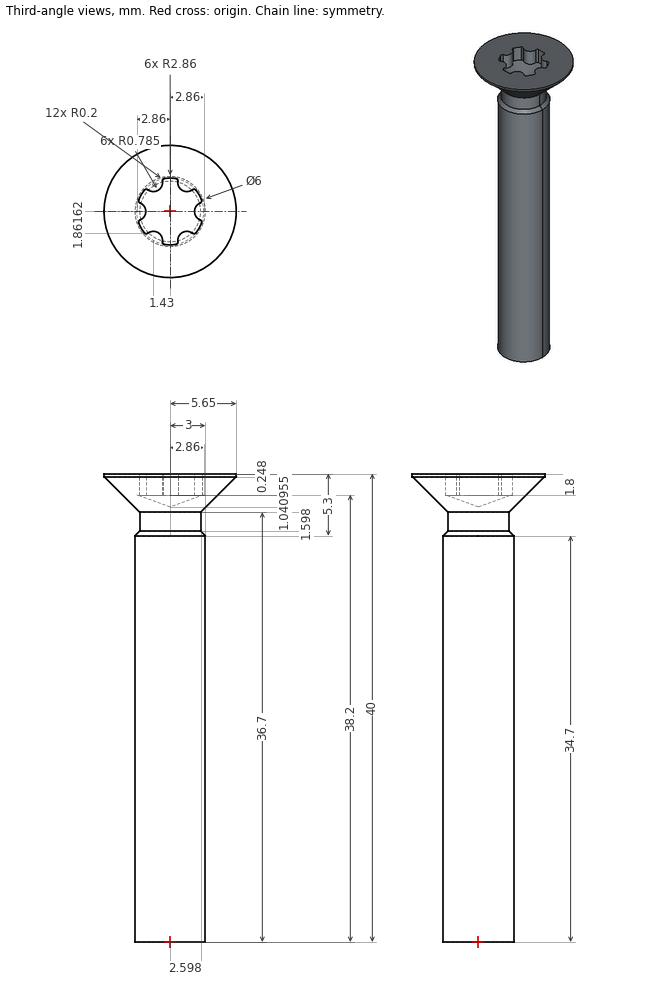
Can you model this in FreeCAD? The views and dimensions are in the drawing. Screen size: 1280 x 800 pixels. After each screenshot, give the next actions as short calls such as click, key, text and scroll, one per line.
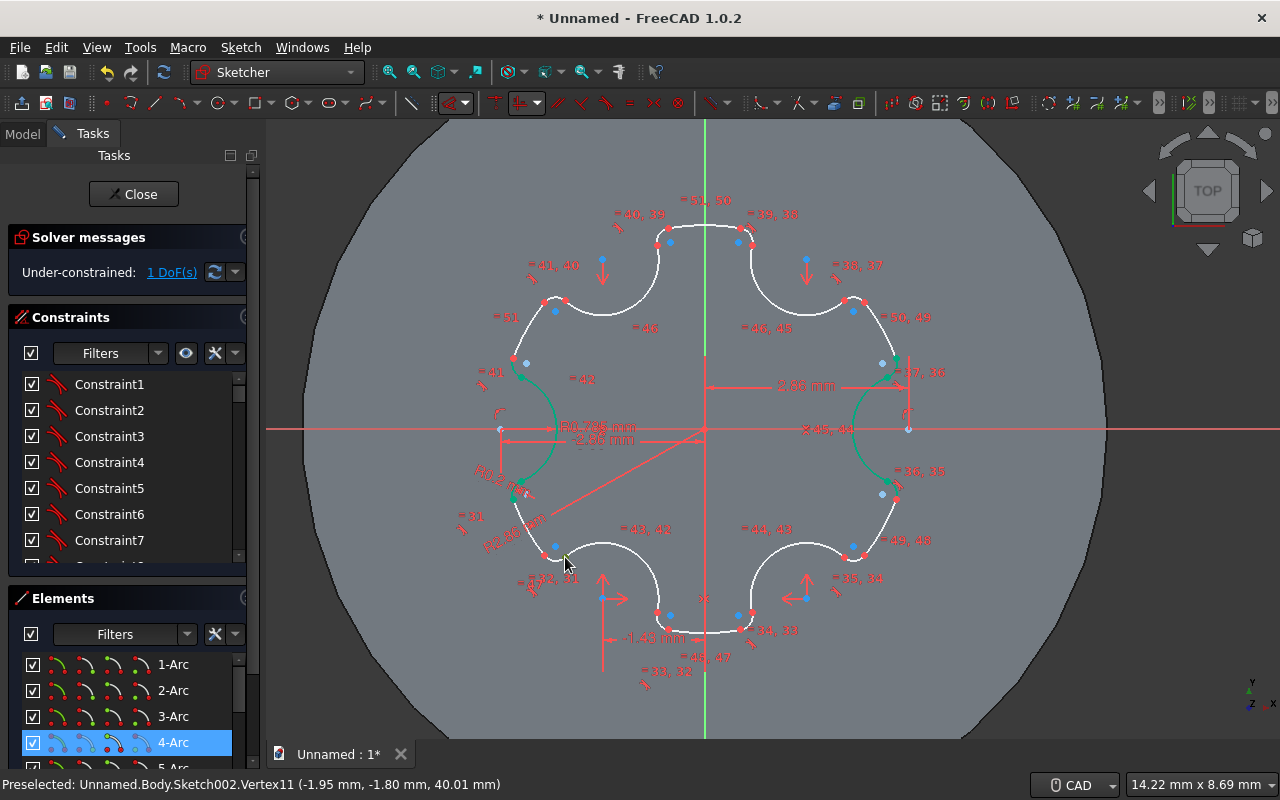
click(468, 104)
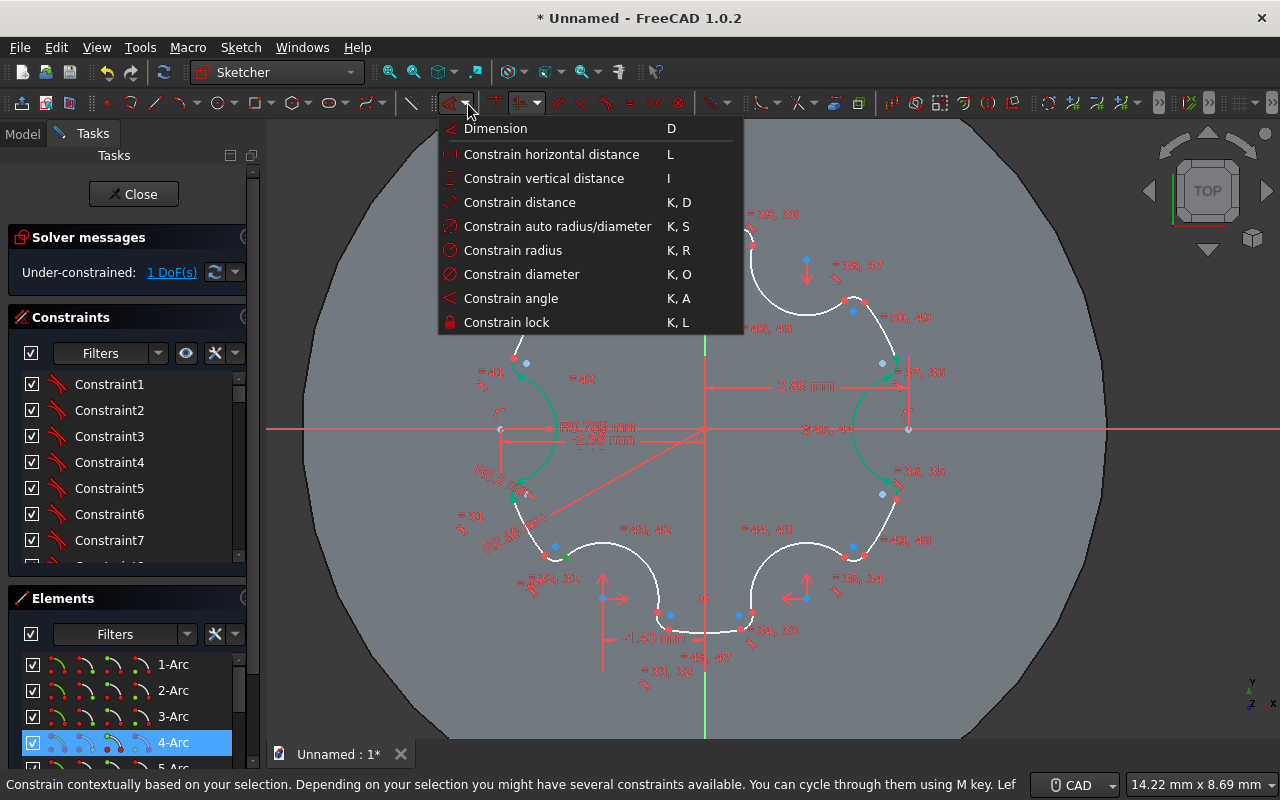
click(591, 178)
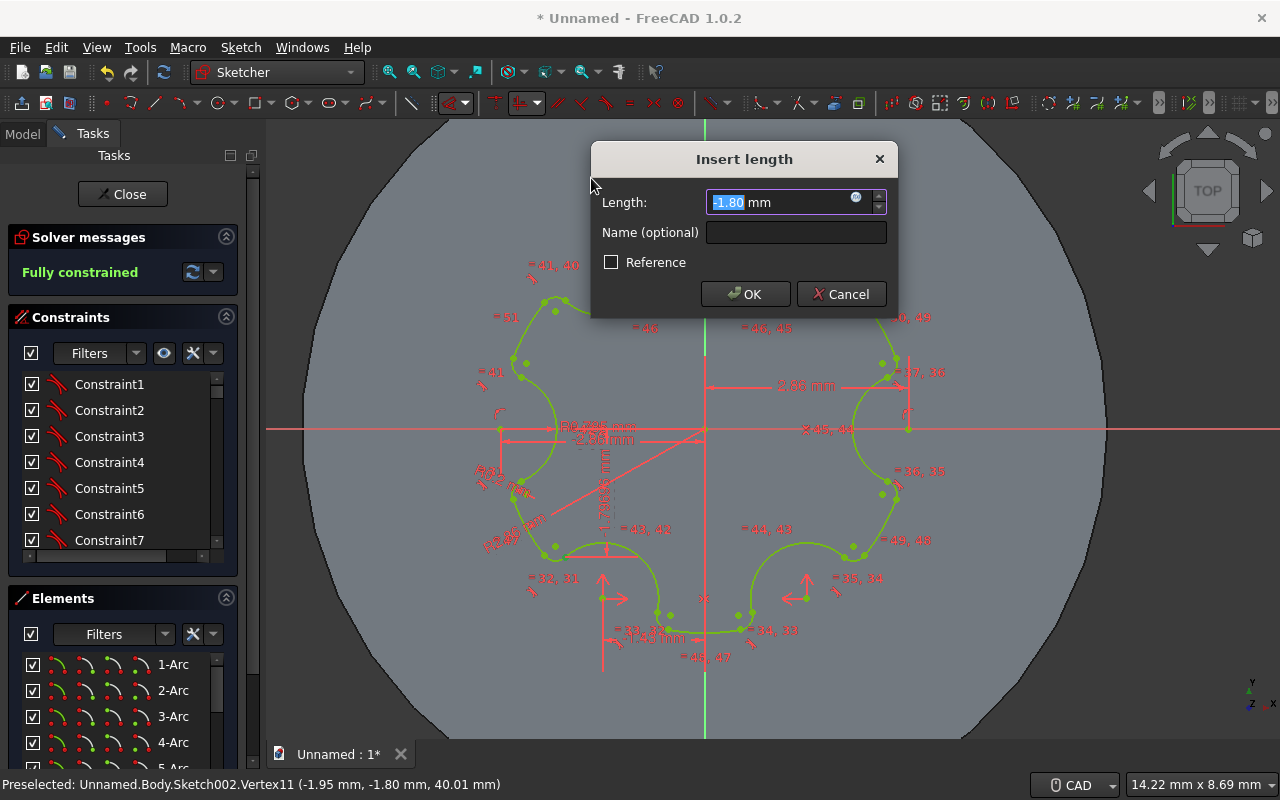
text(-1.86162)
key(Return)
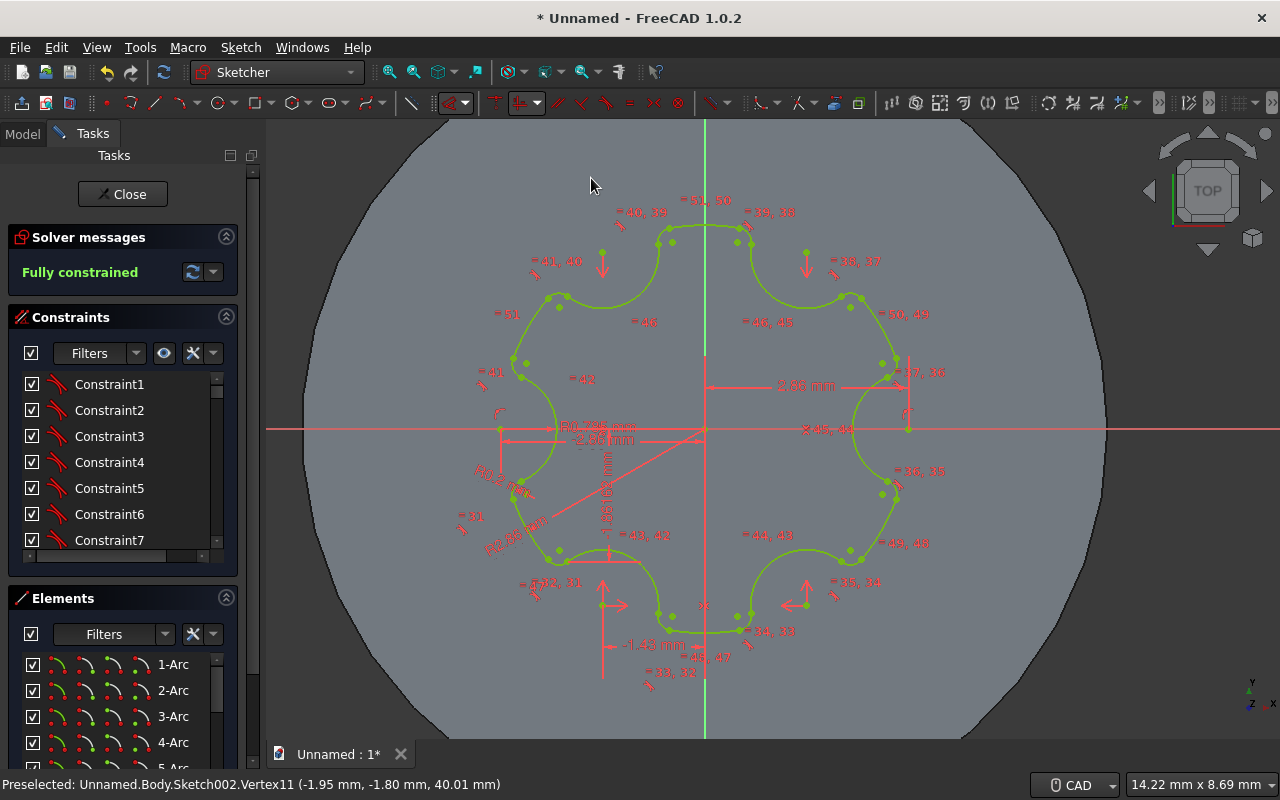
click(123, 194)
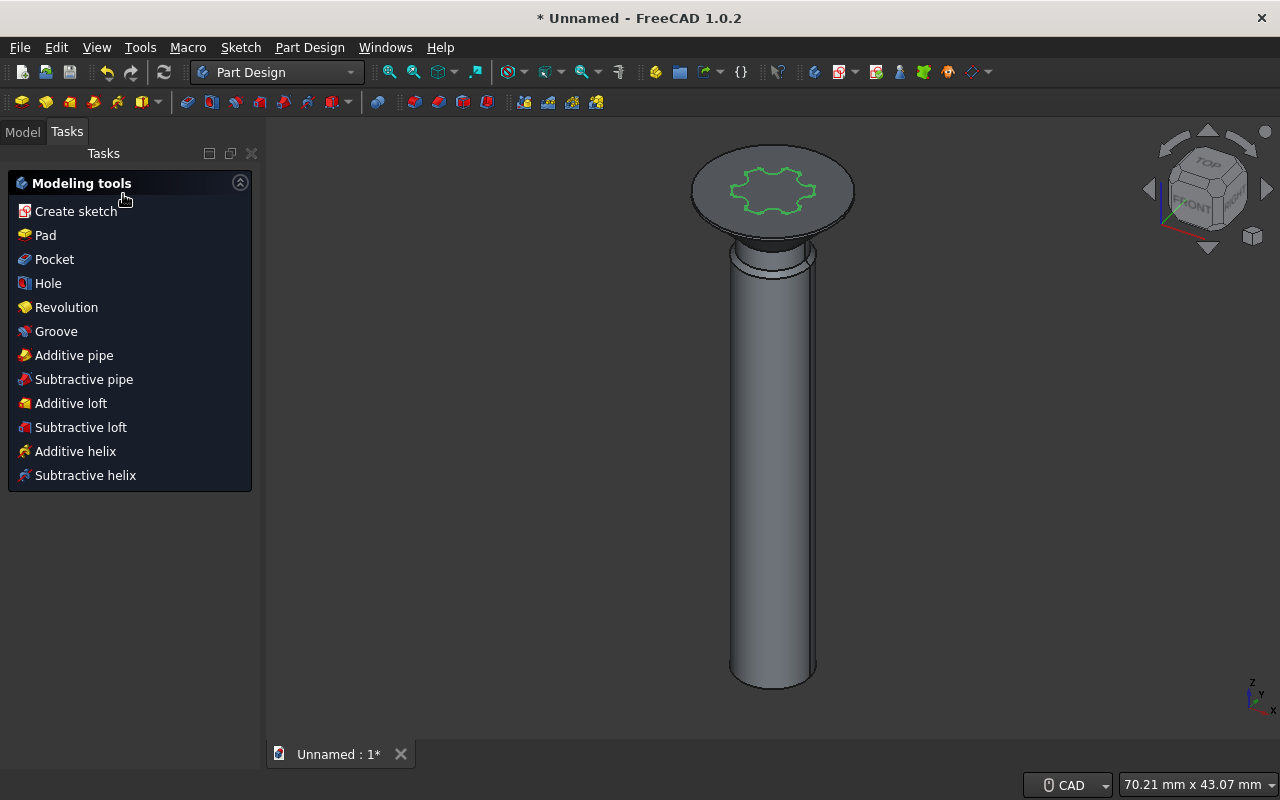
click(188, 102)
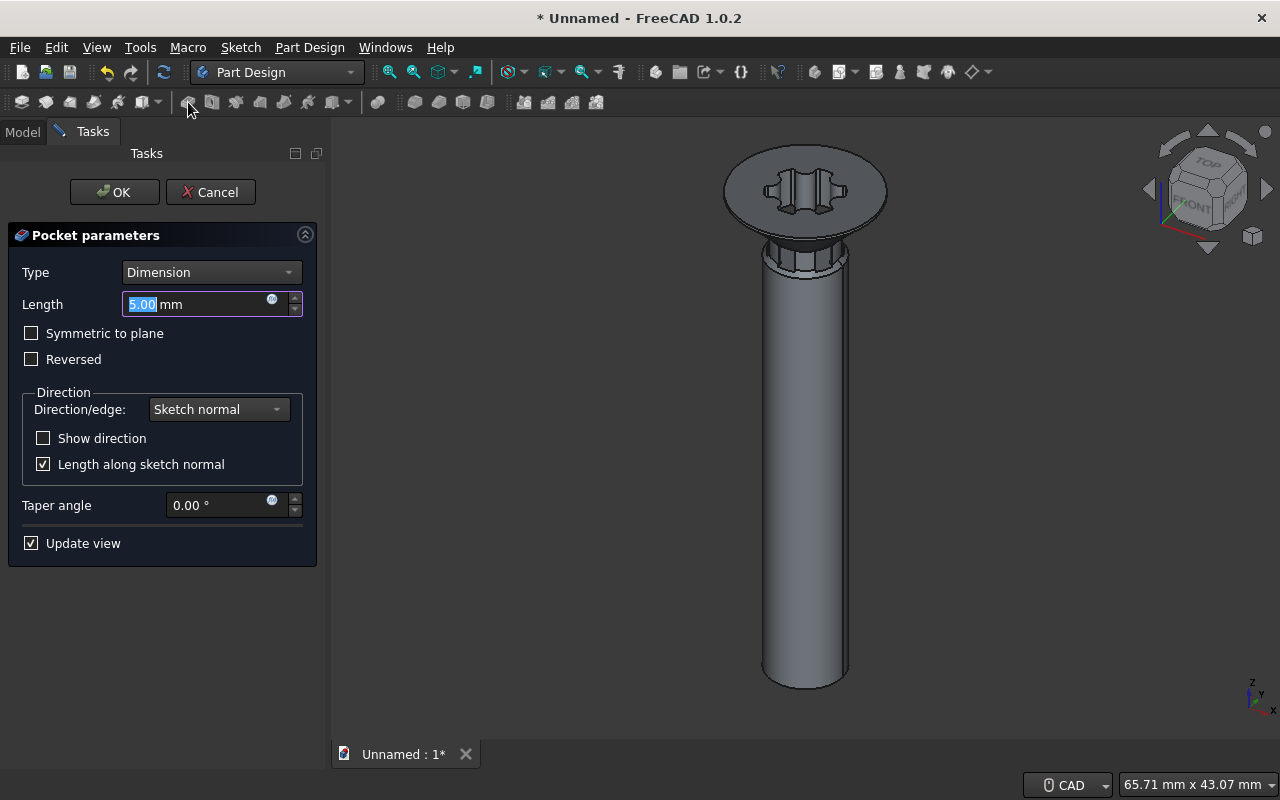
text(1.8)
key(Tab)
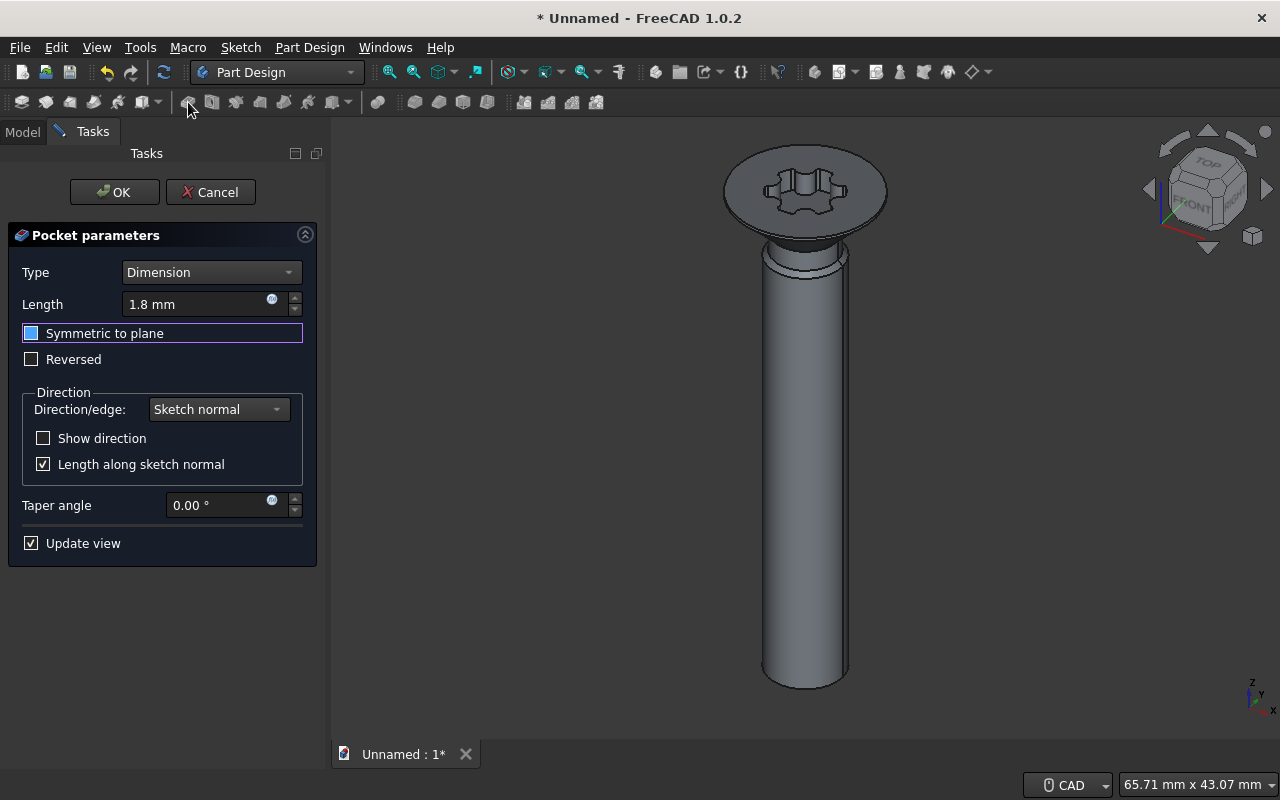
click(115, 192)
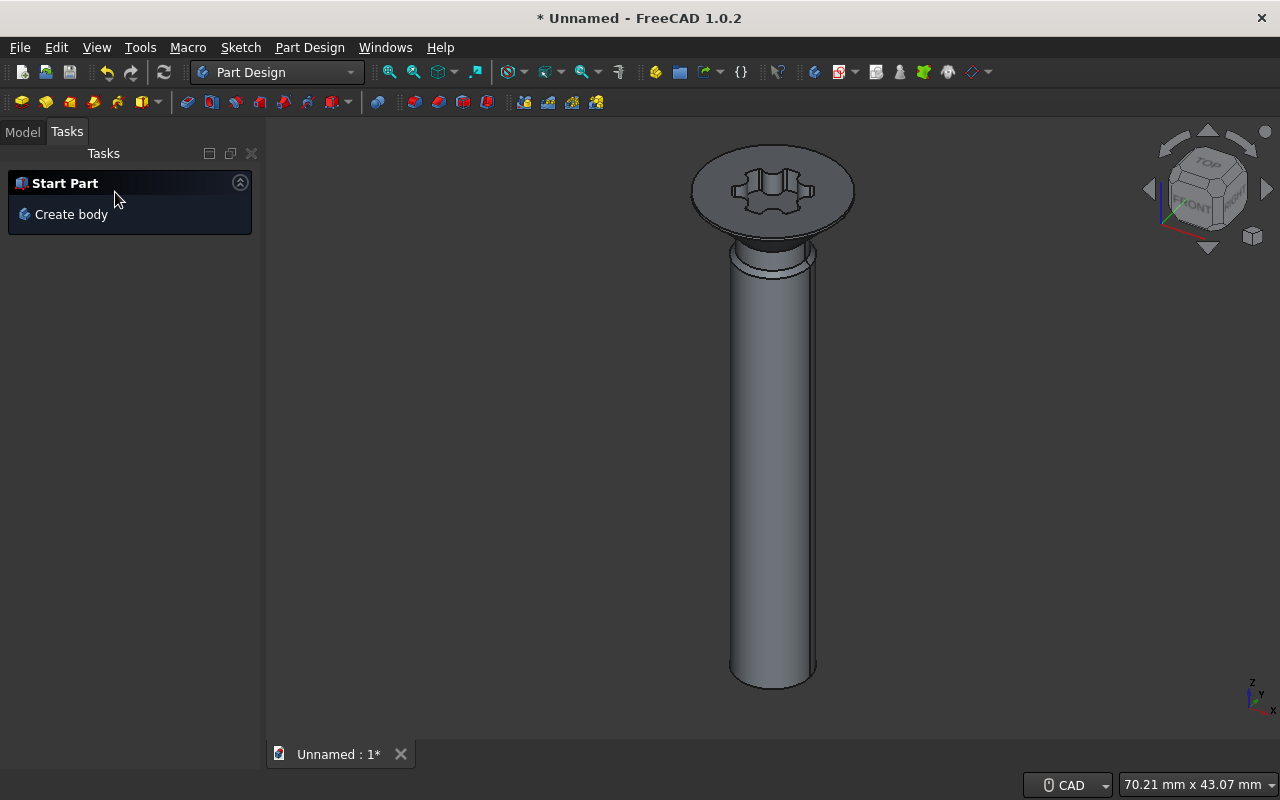
click(840, 72)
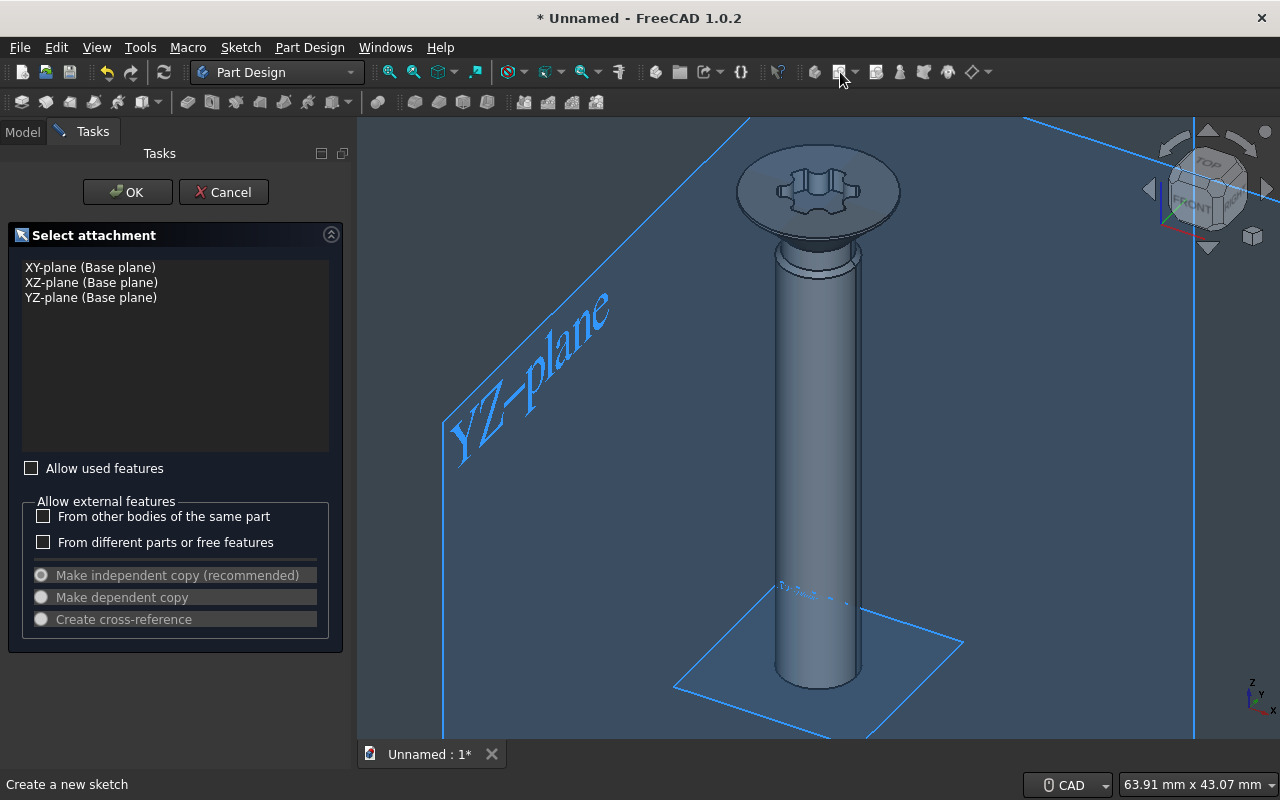
click(82, 282)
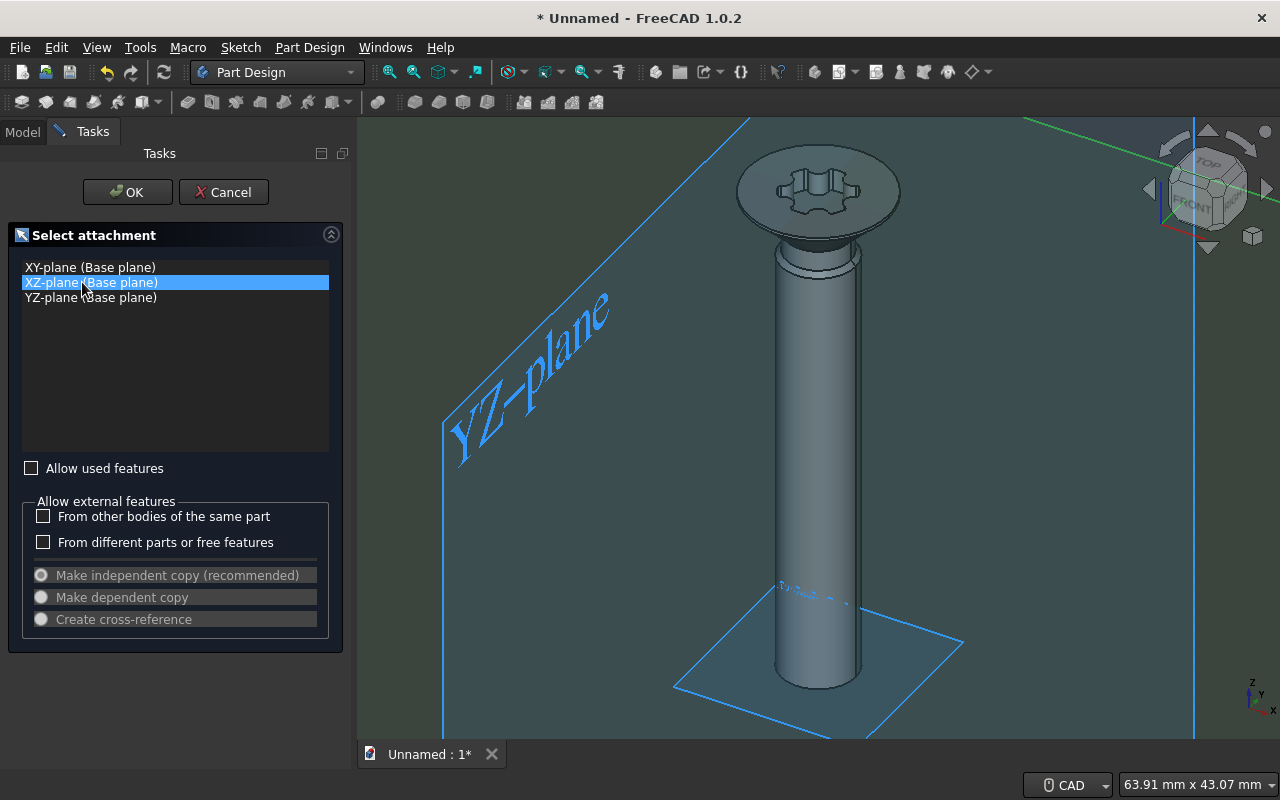
click(128, 192)